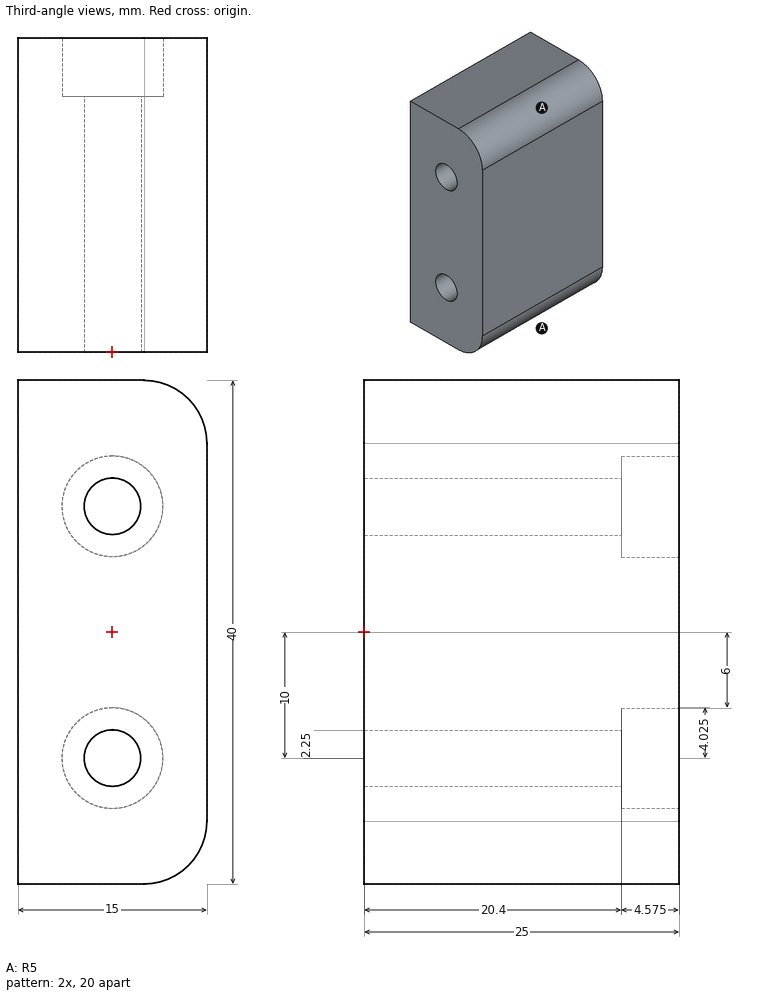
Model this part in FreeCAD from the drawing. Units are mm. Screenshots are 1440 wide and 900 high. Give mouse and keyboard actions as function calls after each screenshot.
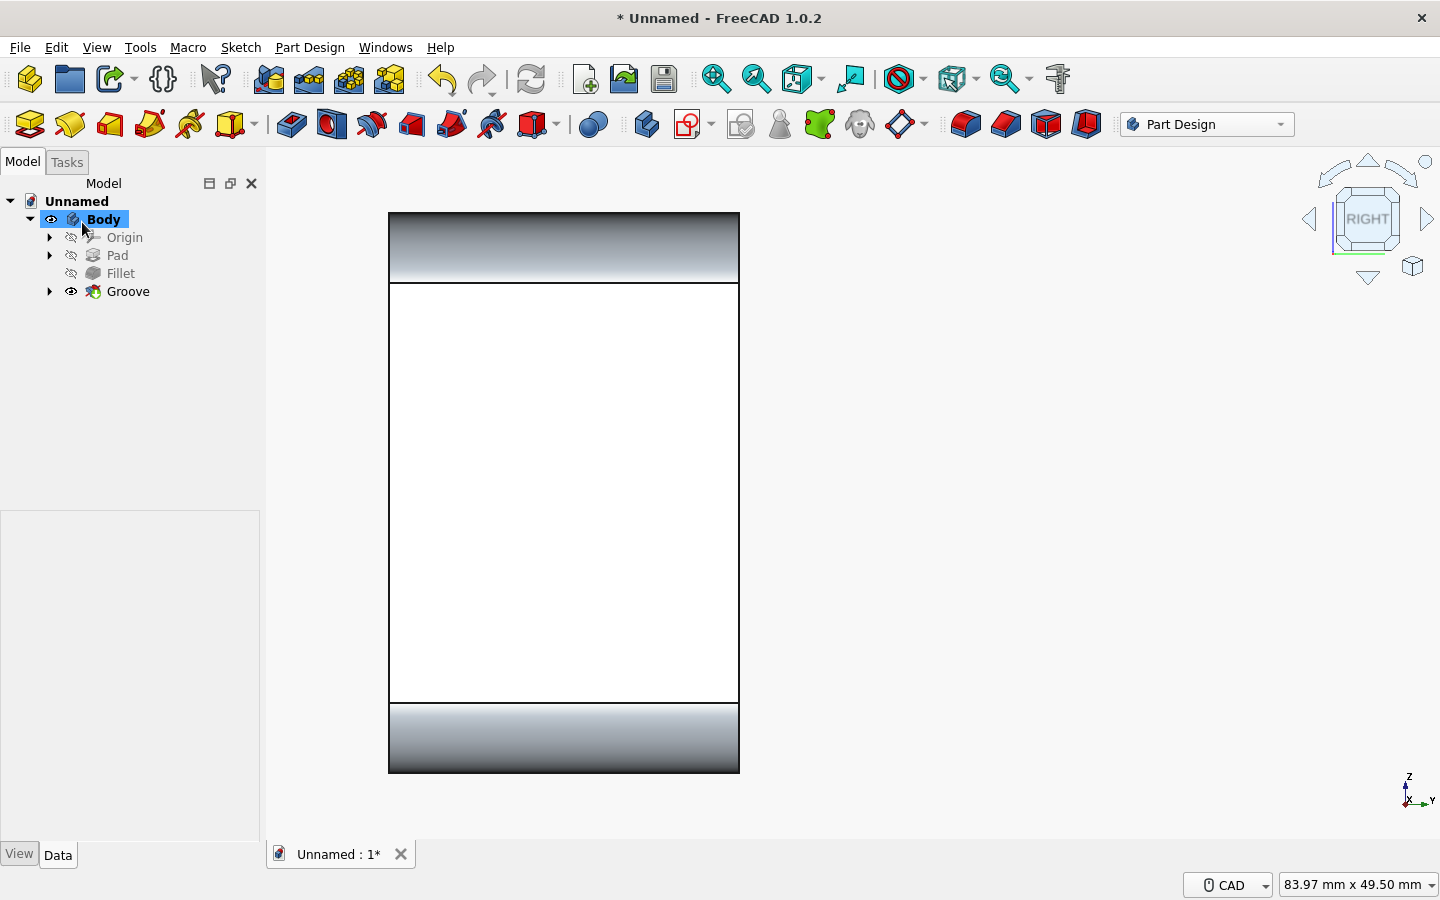
click(116, 291)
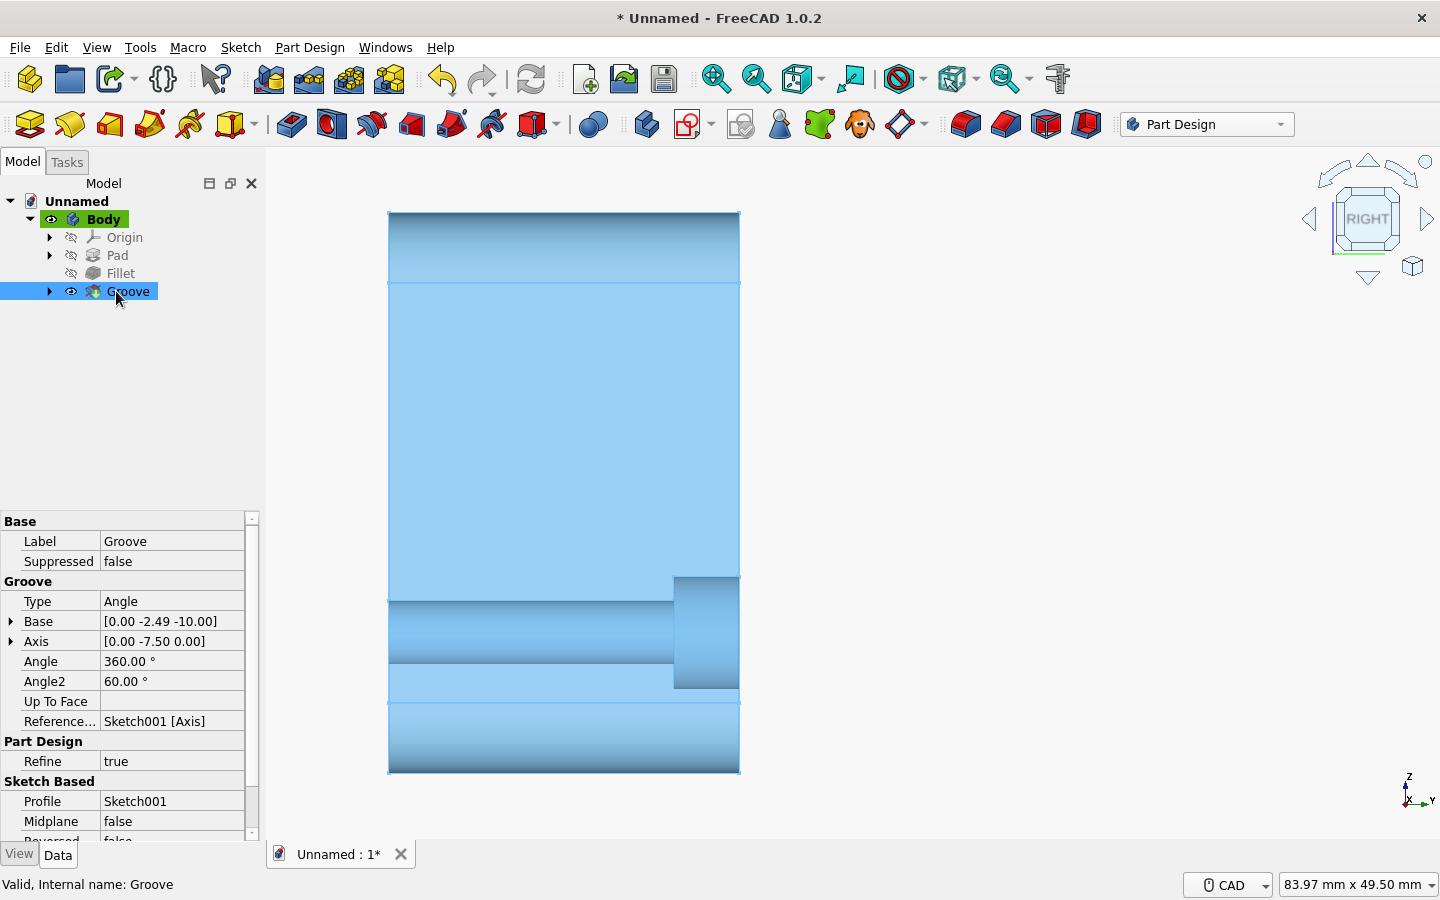
click(310, 80)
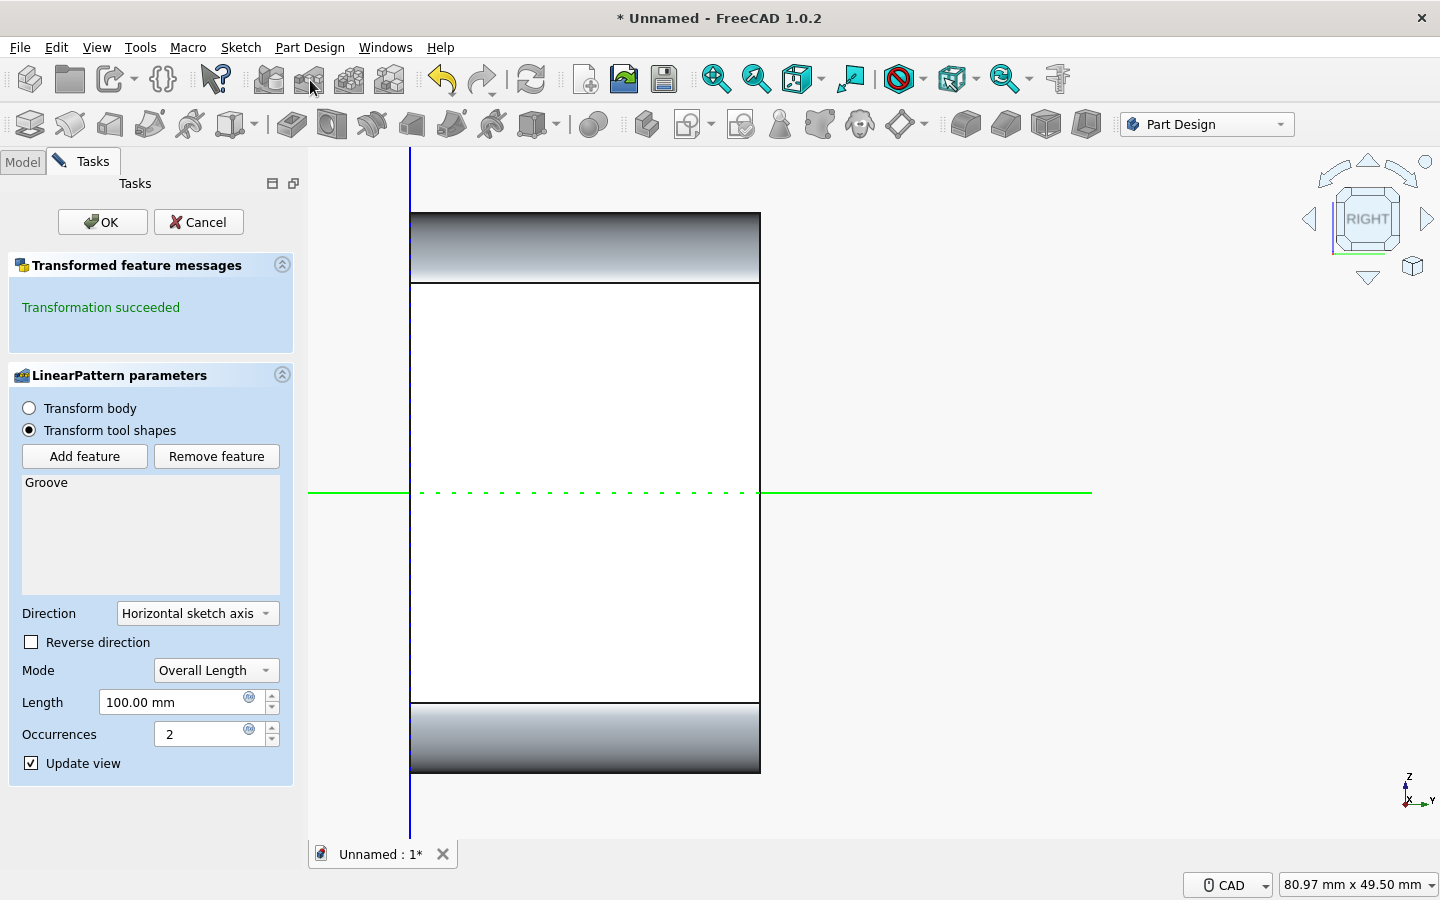
click(198, 614)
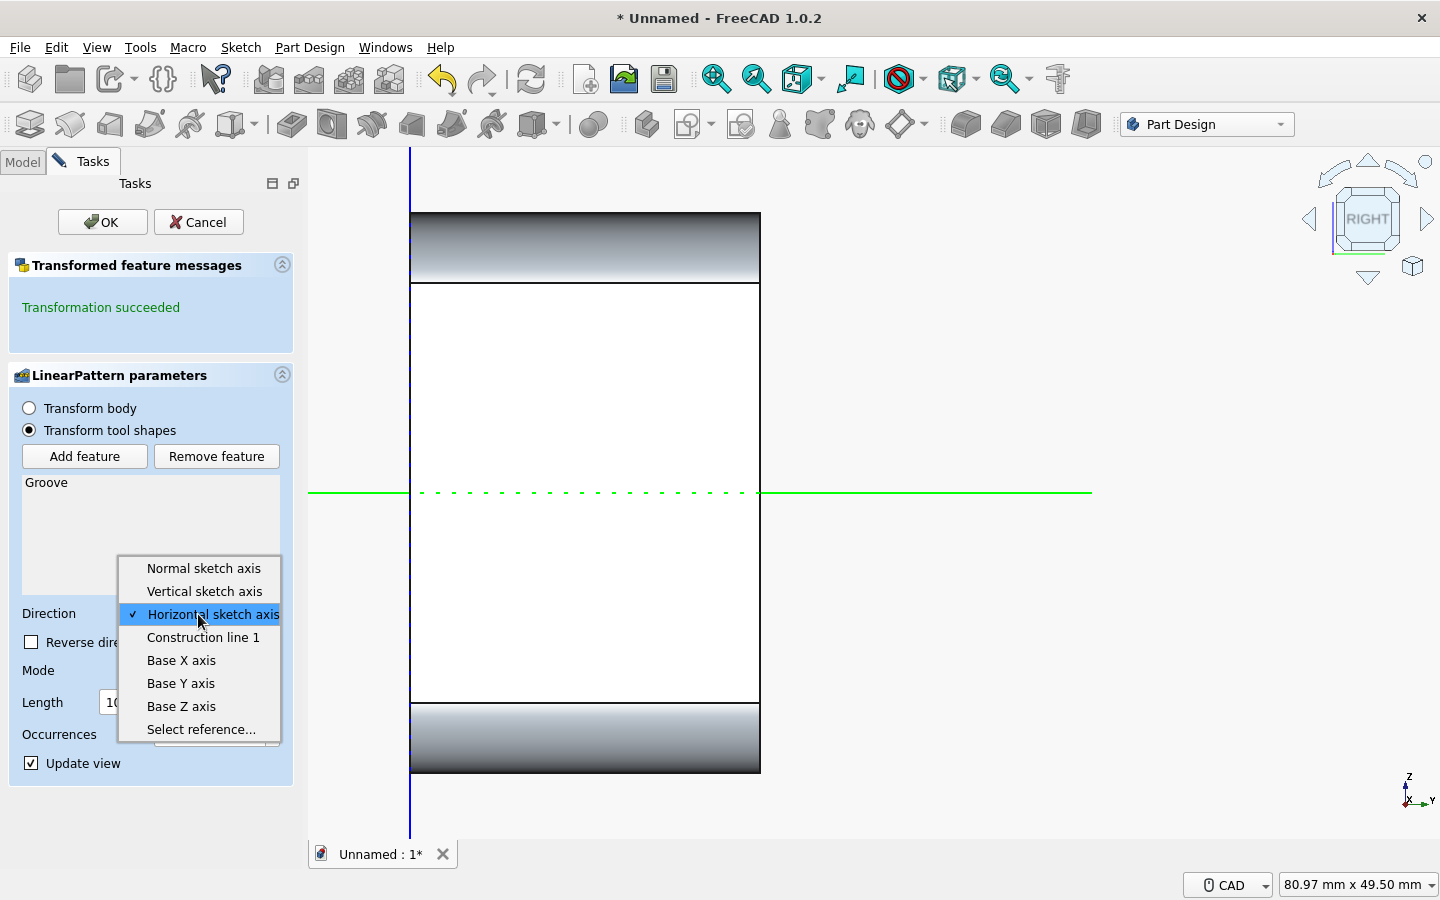
click(198, 706)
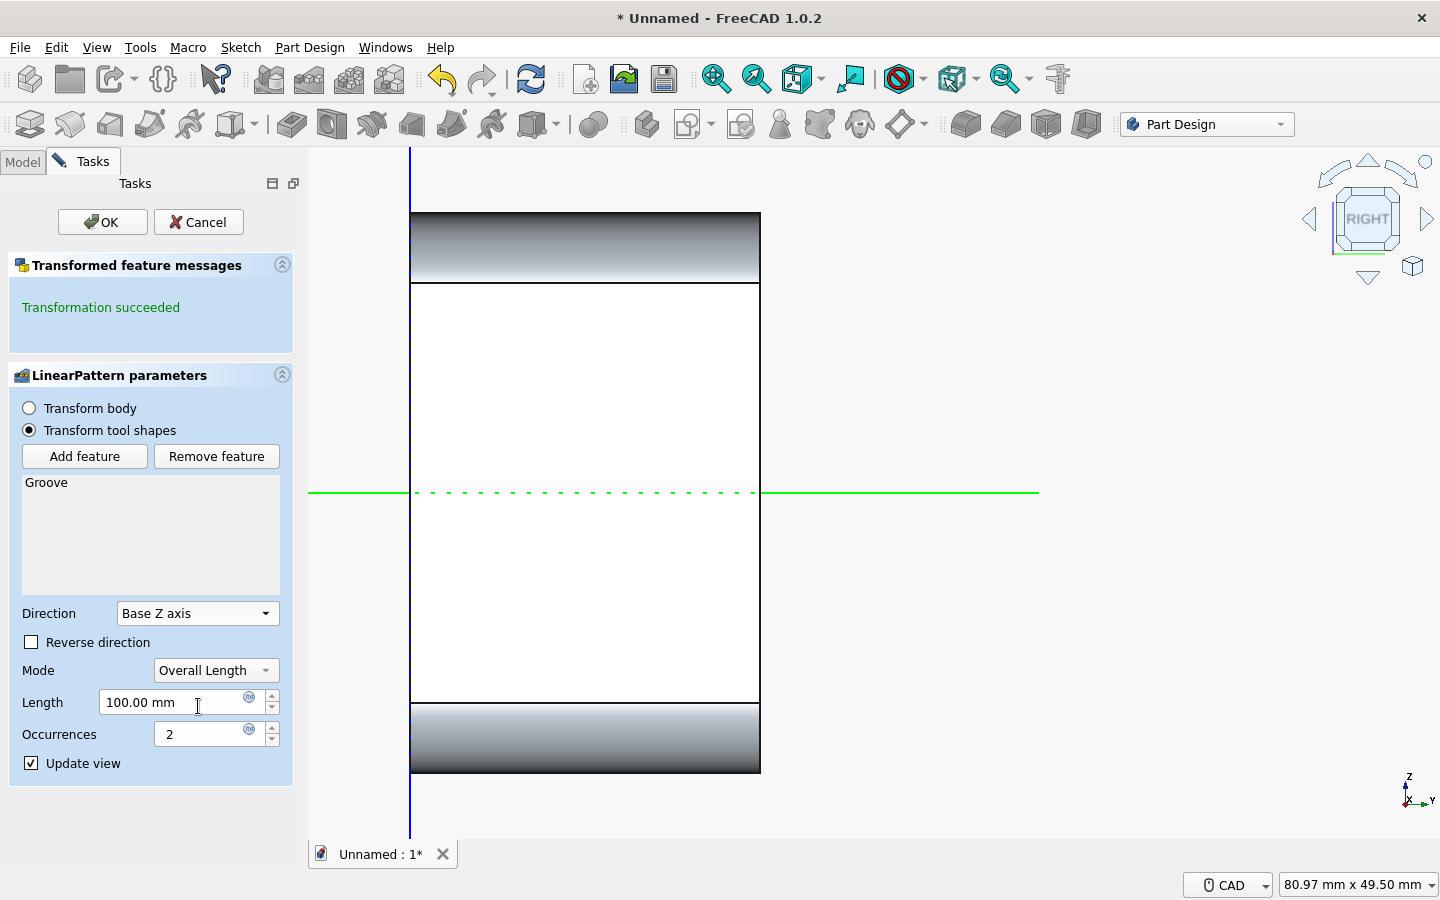
click(217, 670)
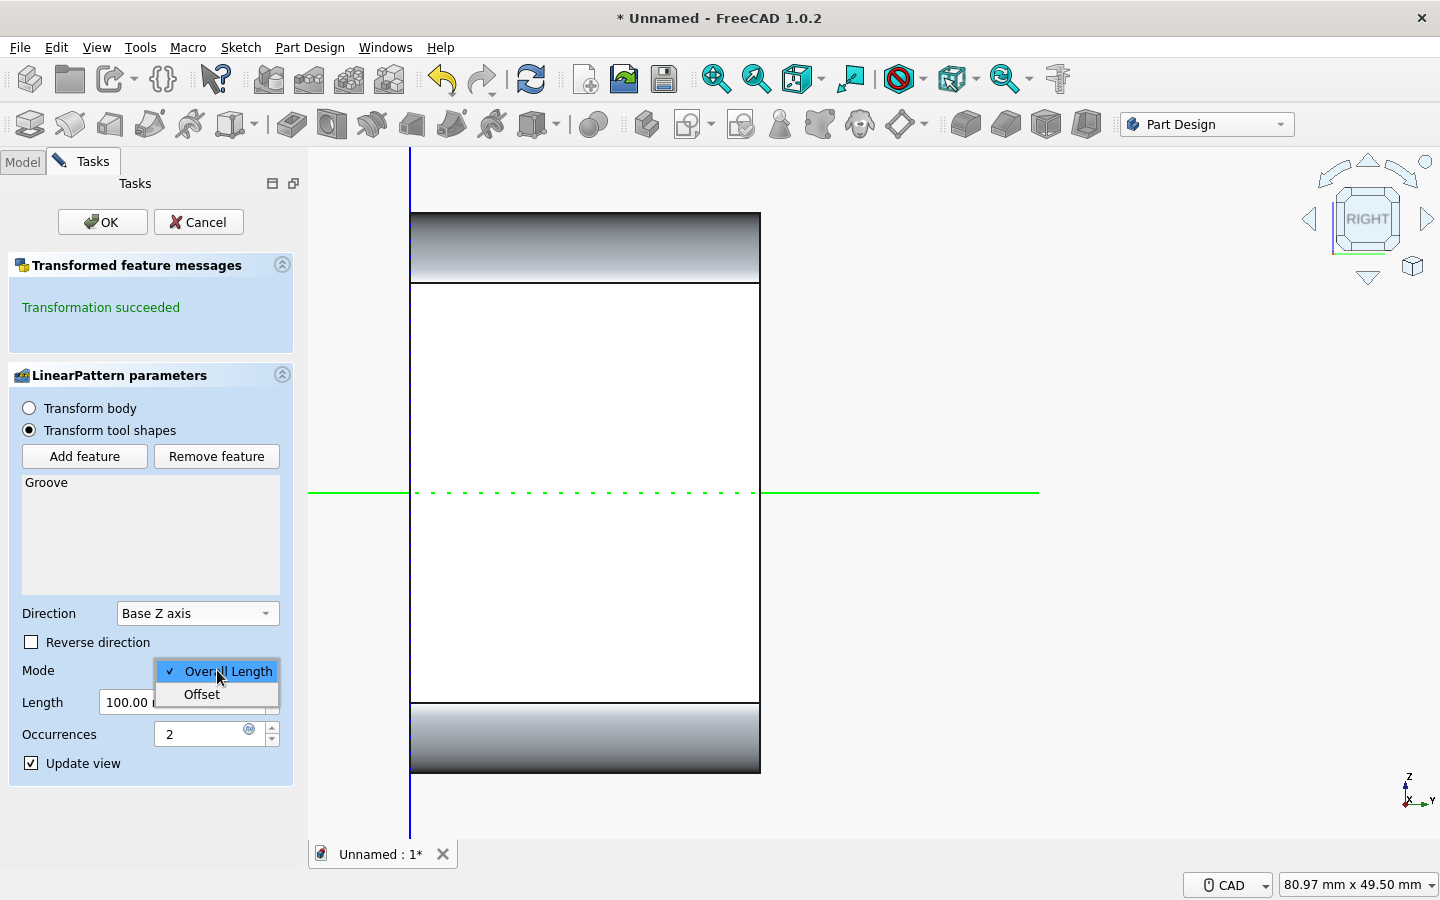
click(216, 694)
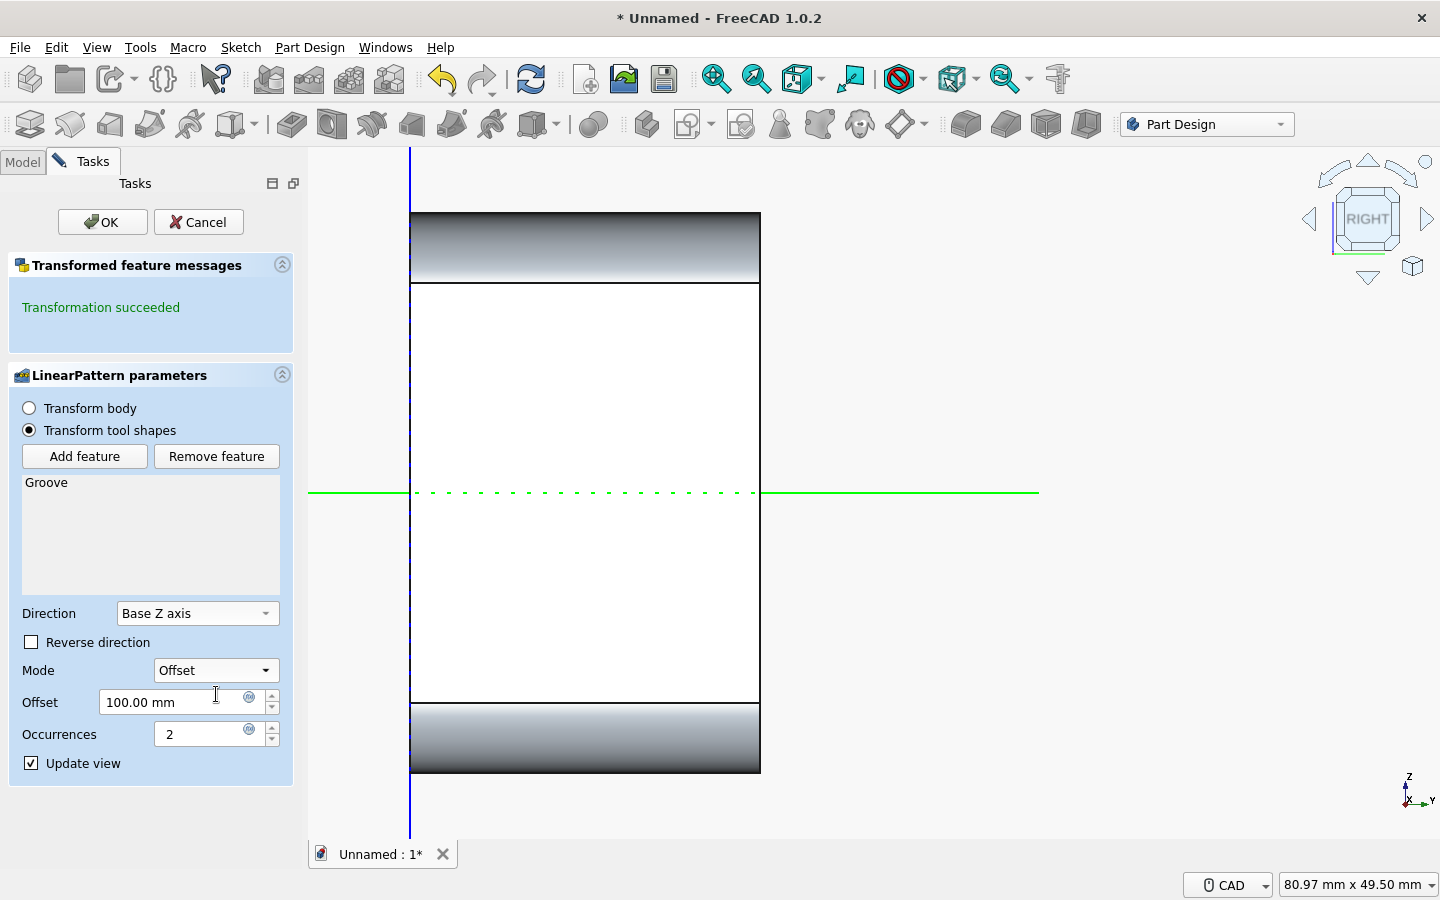
triple_click(182, 702)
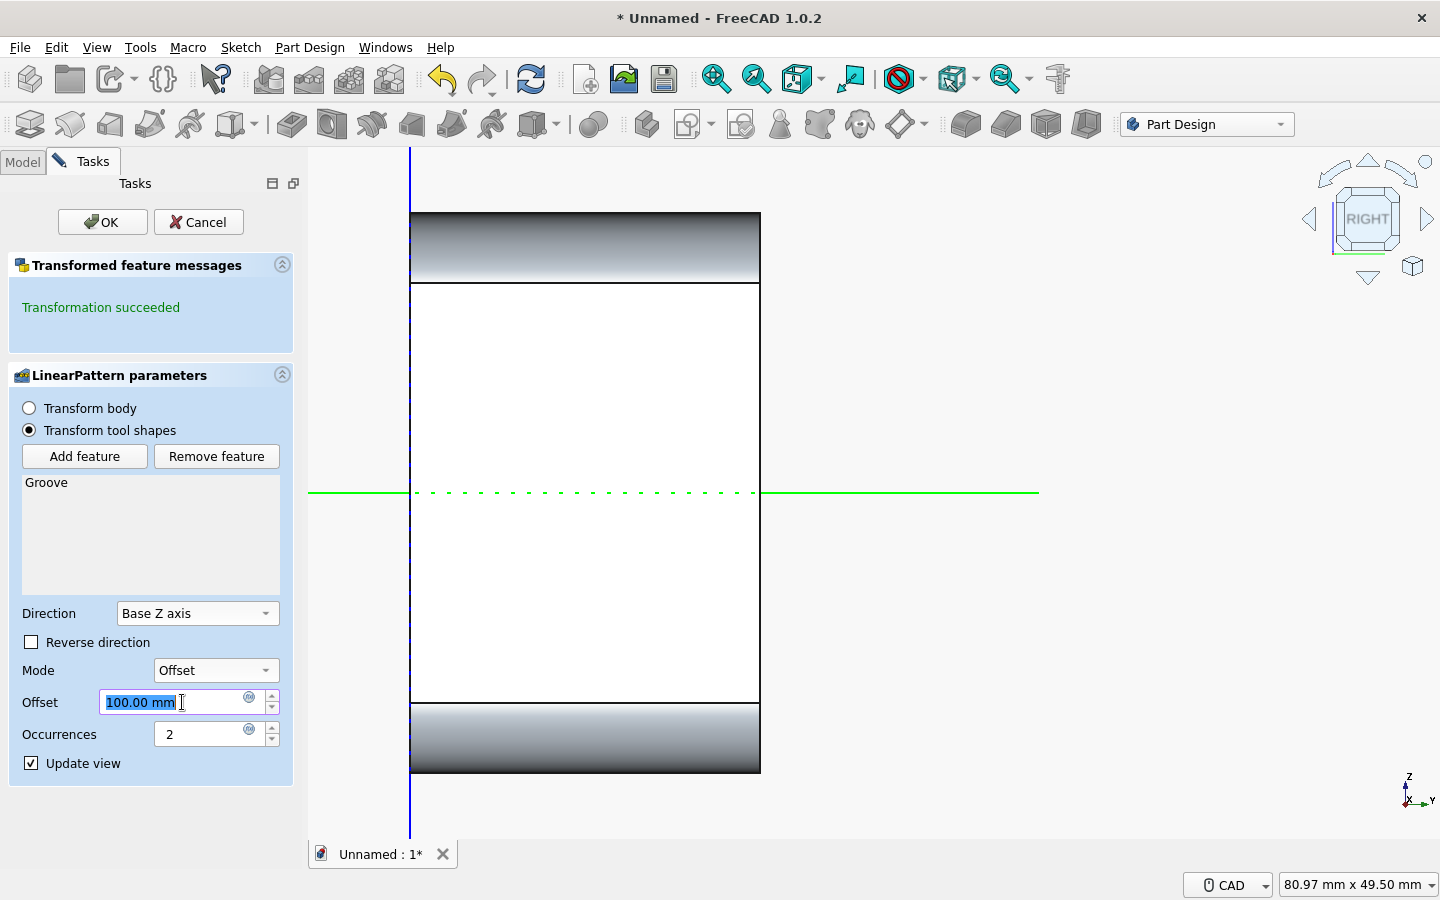
text(20)
key(Tab)